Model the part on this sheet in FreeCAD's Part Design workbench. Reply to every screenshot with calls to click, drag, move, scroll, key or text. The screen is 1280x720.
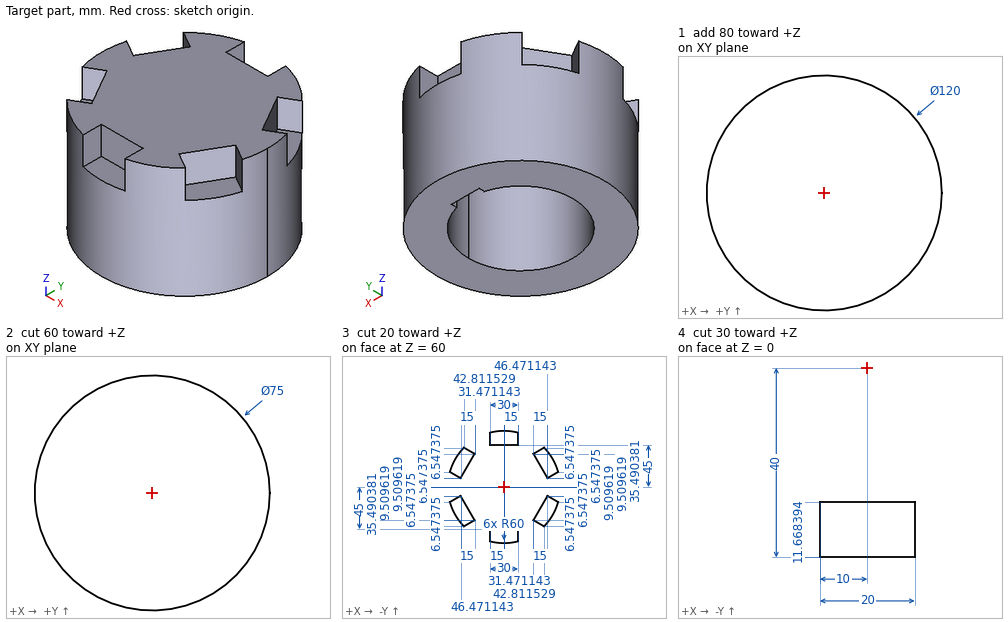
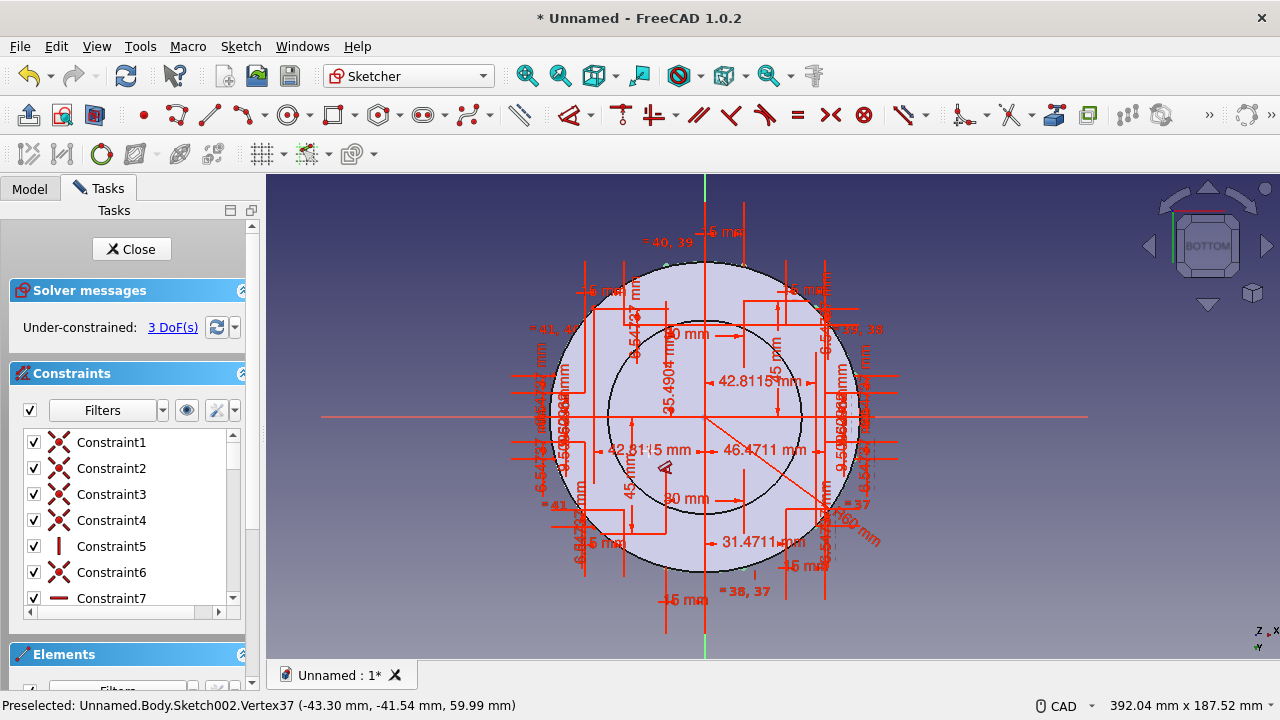
click(624, 325)
click(646, 267)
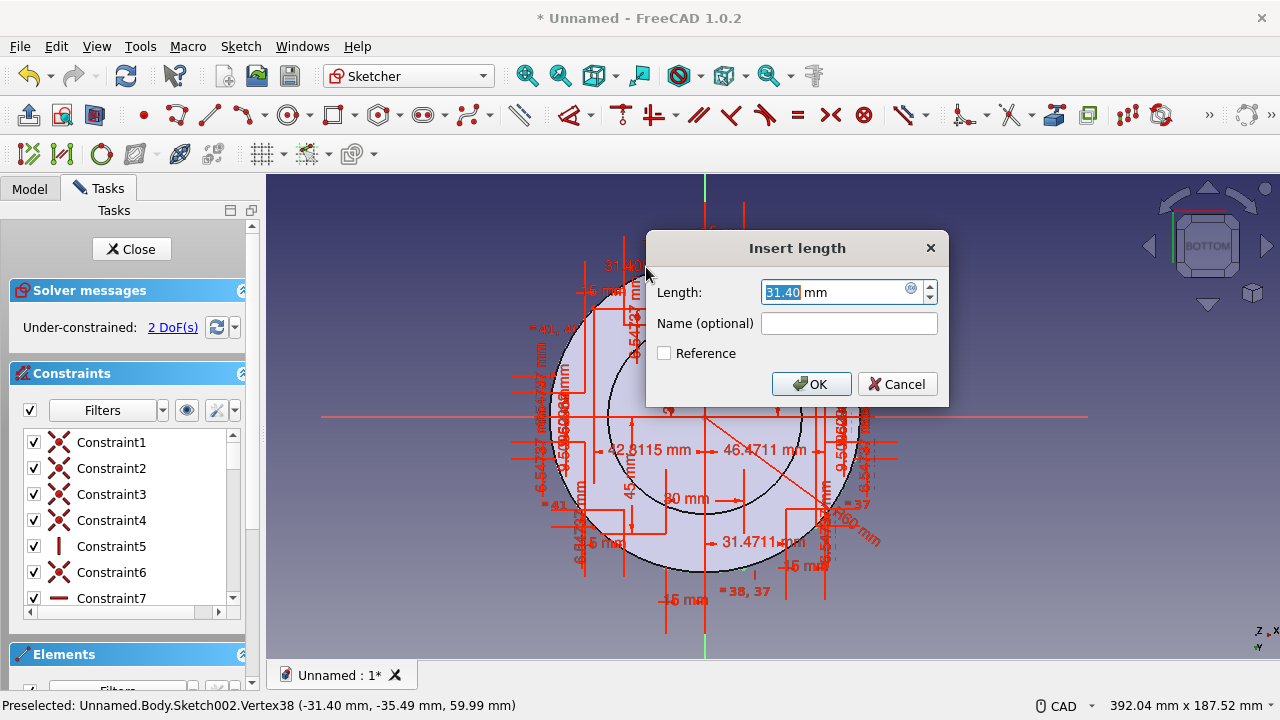
text(31.471143)
key(Return)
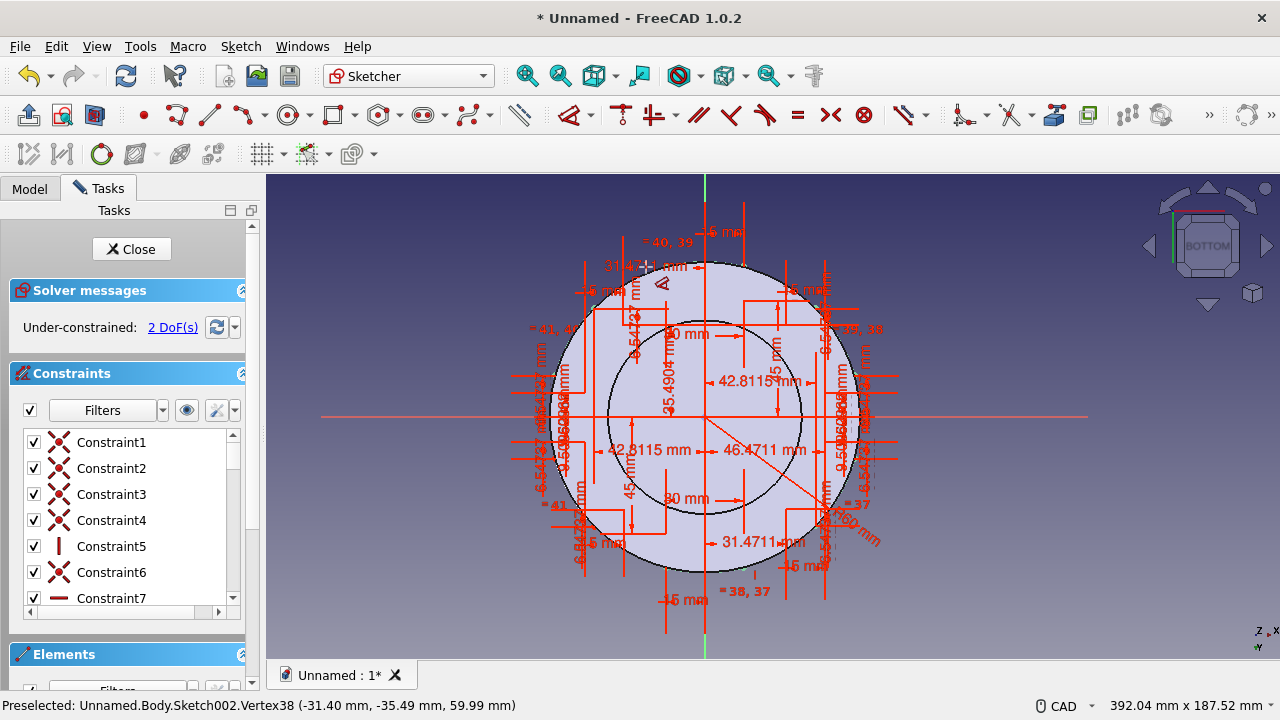
click(585, 442)
click(603, 500)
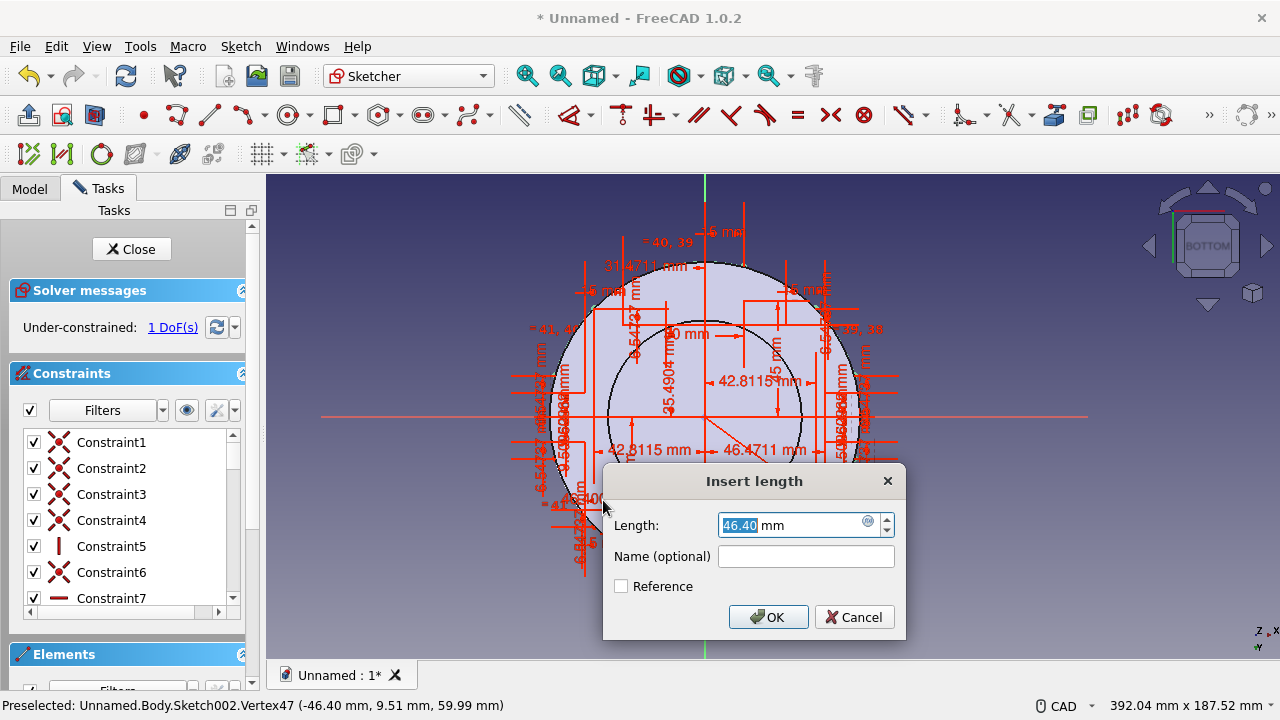
text(46.471143)
key(Return)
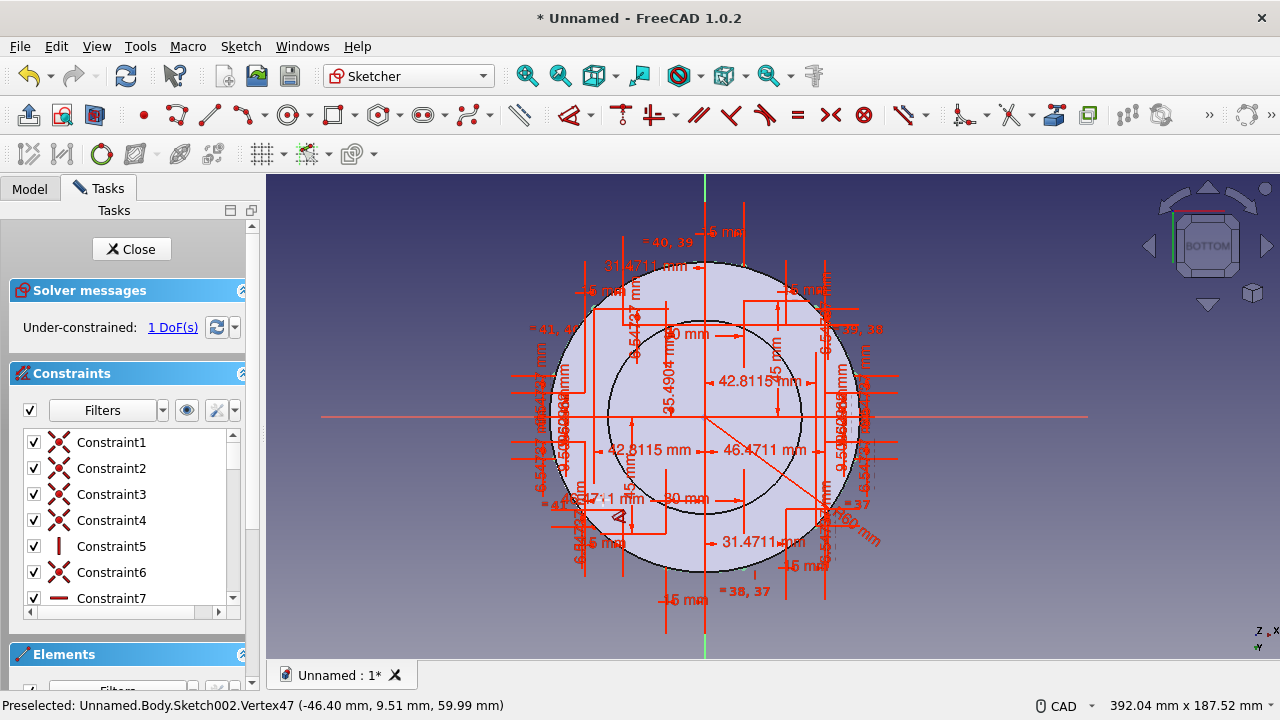
click(623, 510)
click(739, 431)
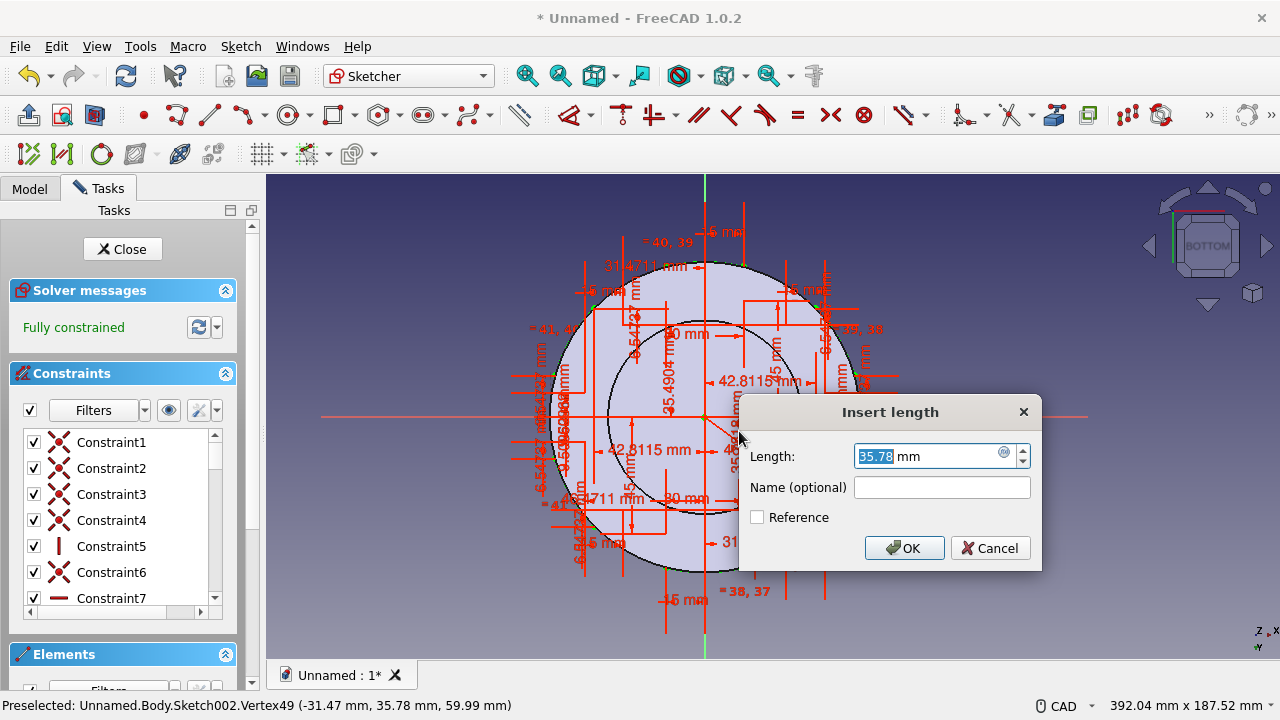
text(35.490381)
key(Return)
key(Escape)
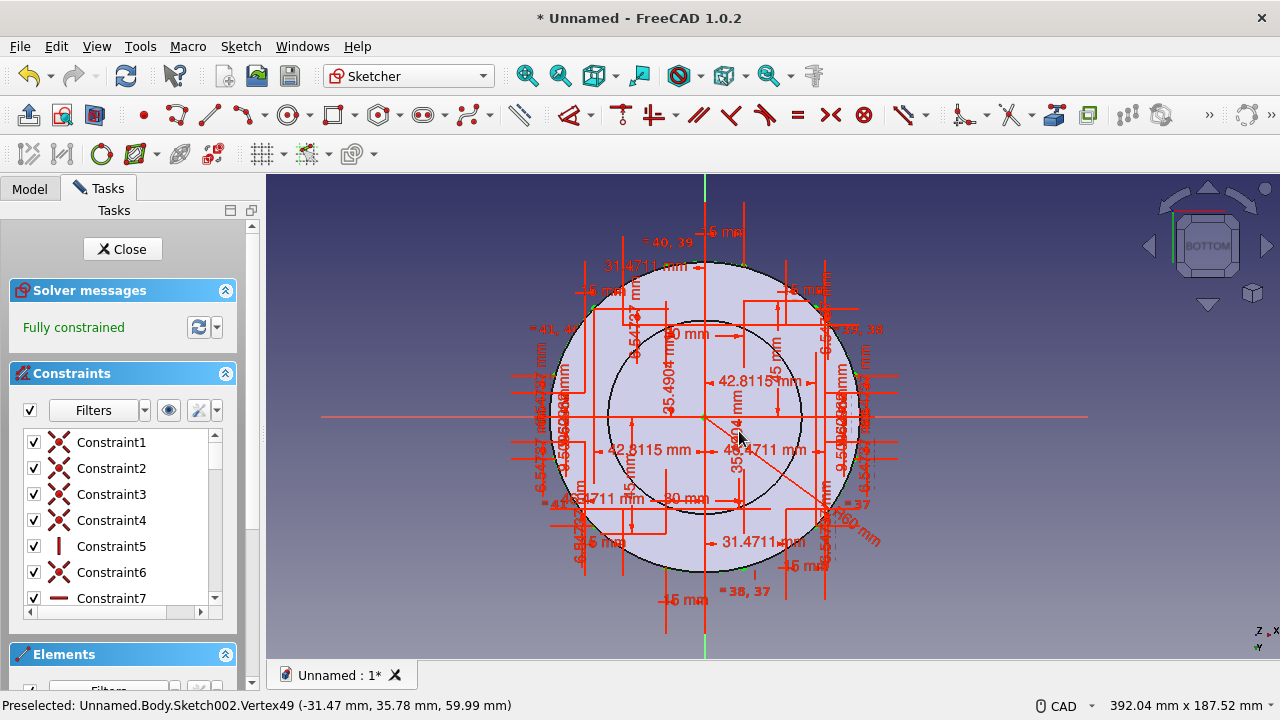
click(123, 249)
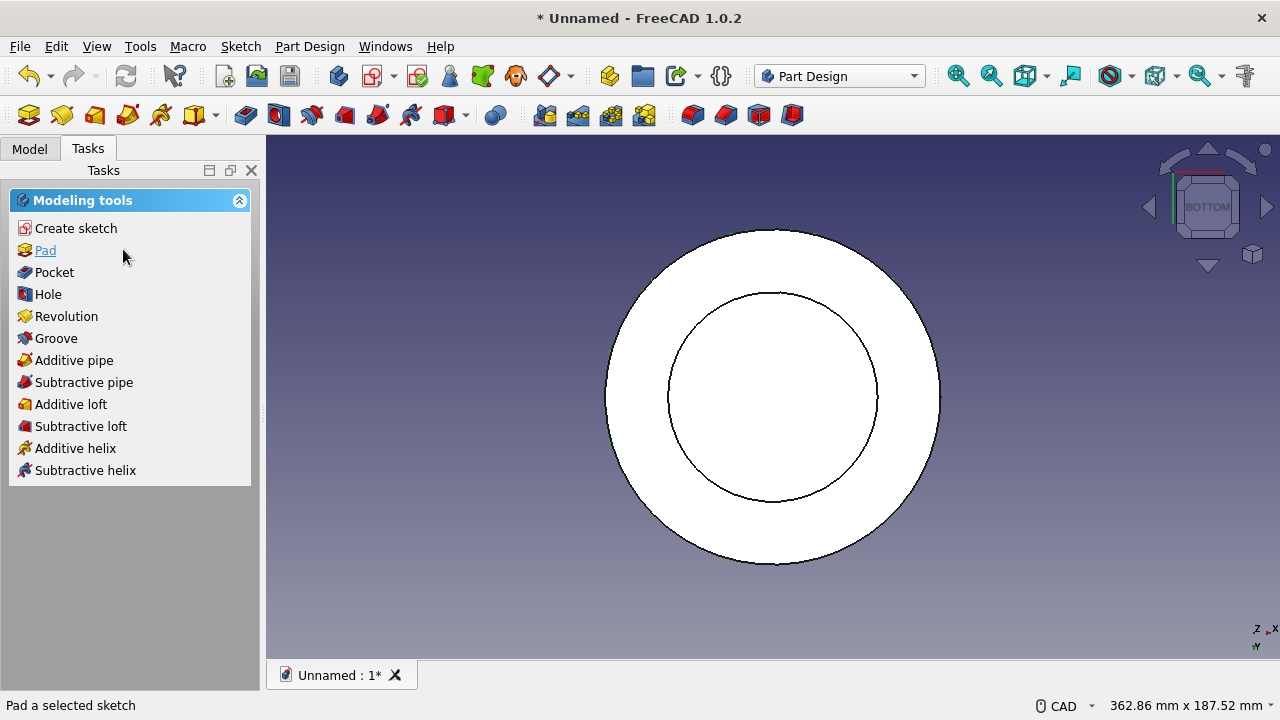
click(246, 116)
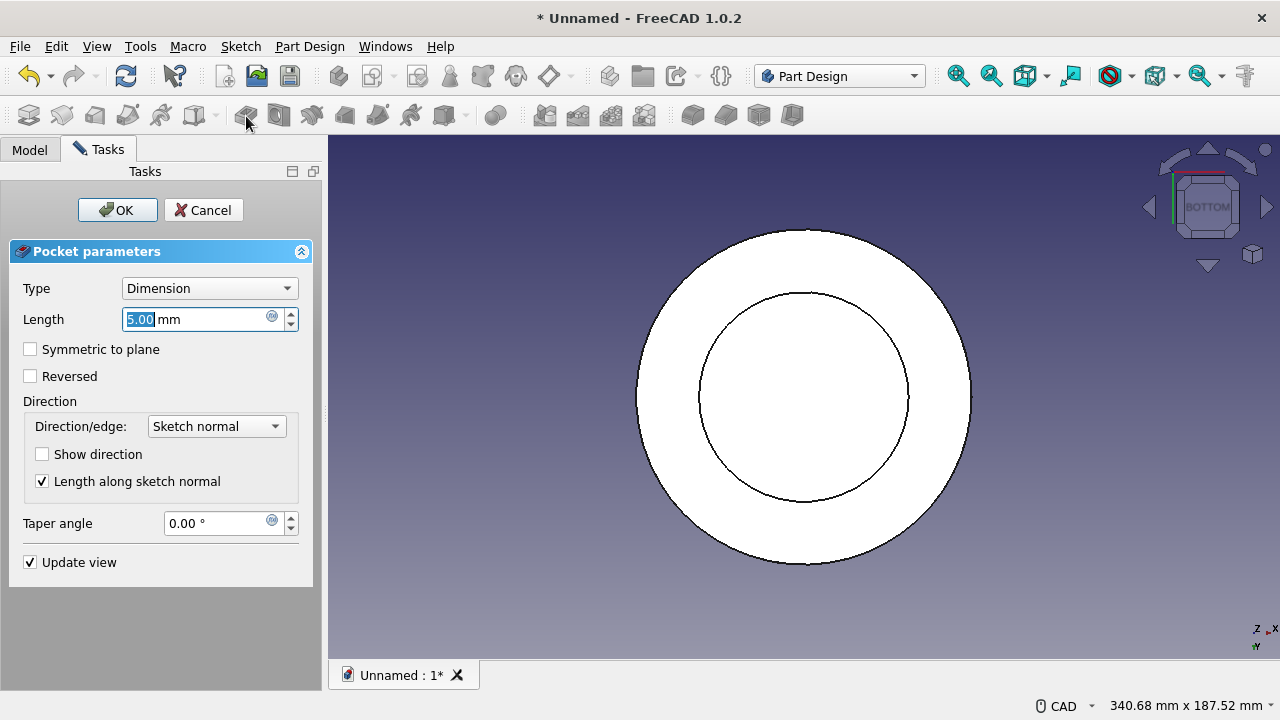
text(20)
key(Tab)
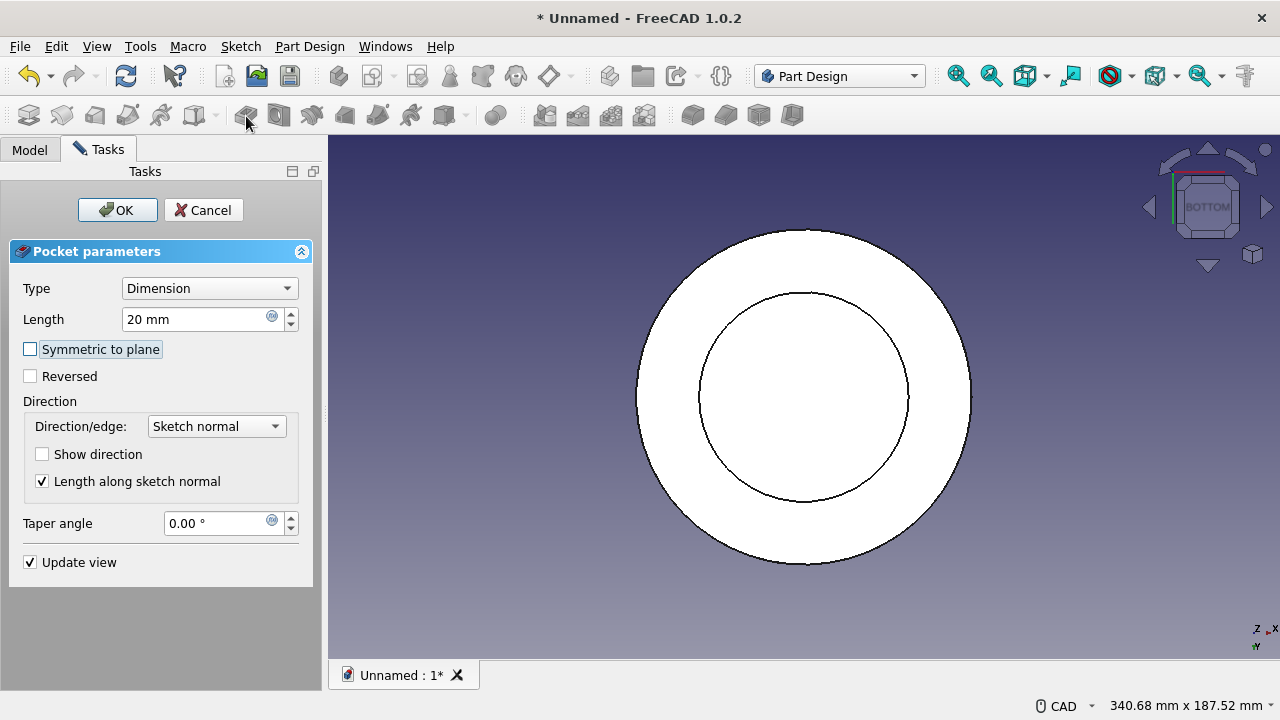
click(118, 210)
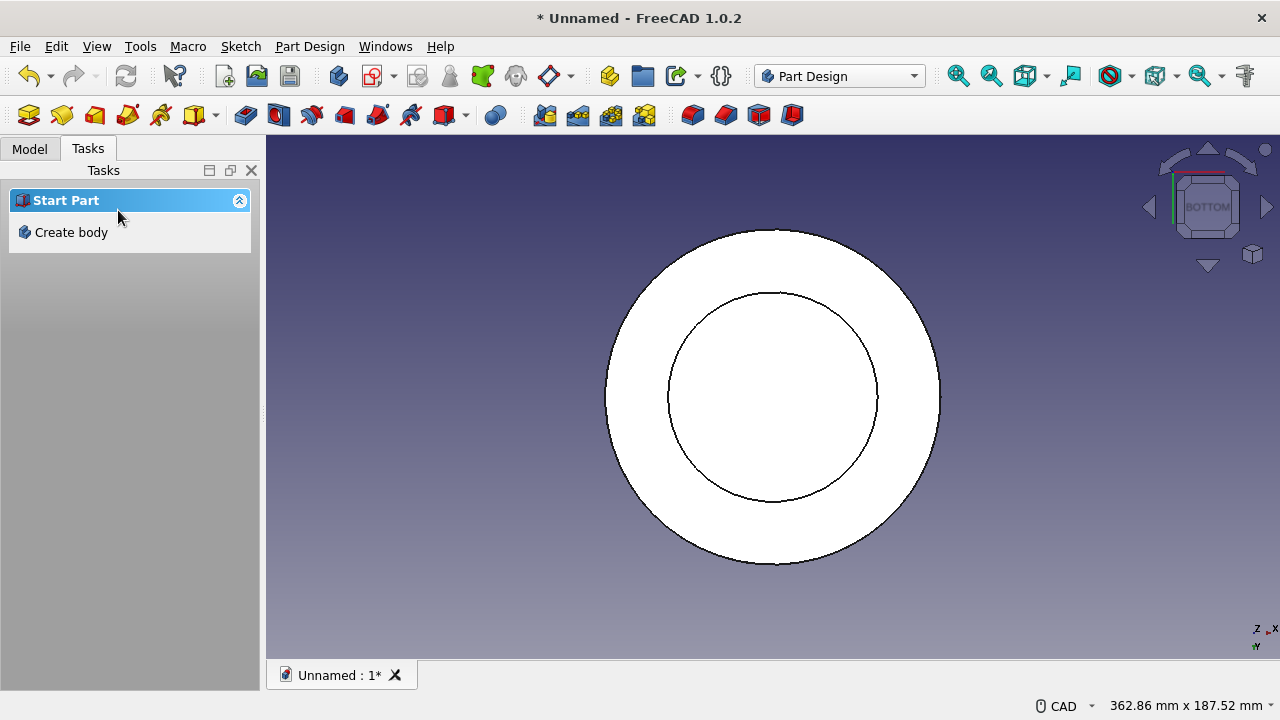
click(869, 492)